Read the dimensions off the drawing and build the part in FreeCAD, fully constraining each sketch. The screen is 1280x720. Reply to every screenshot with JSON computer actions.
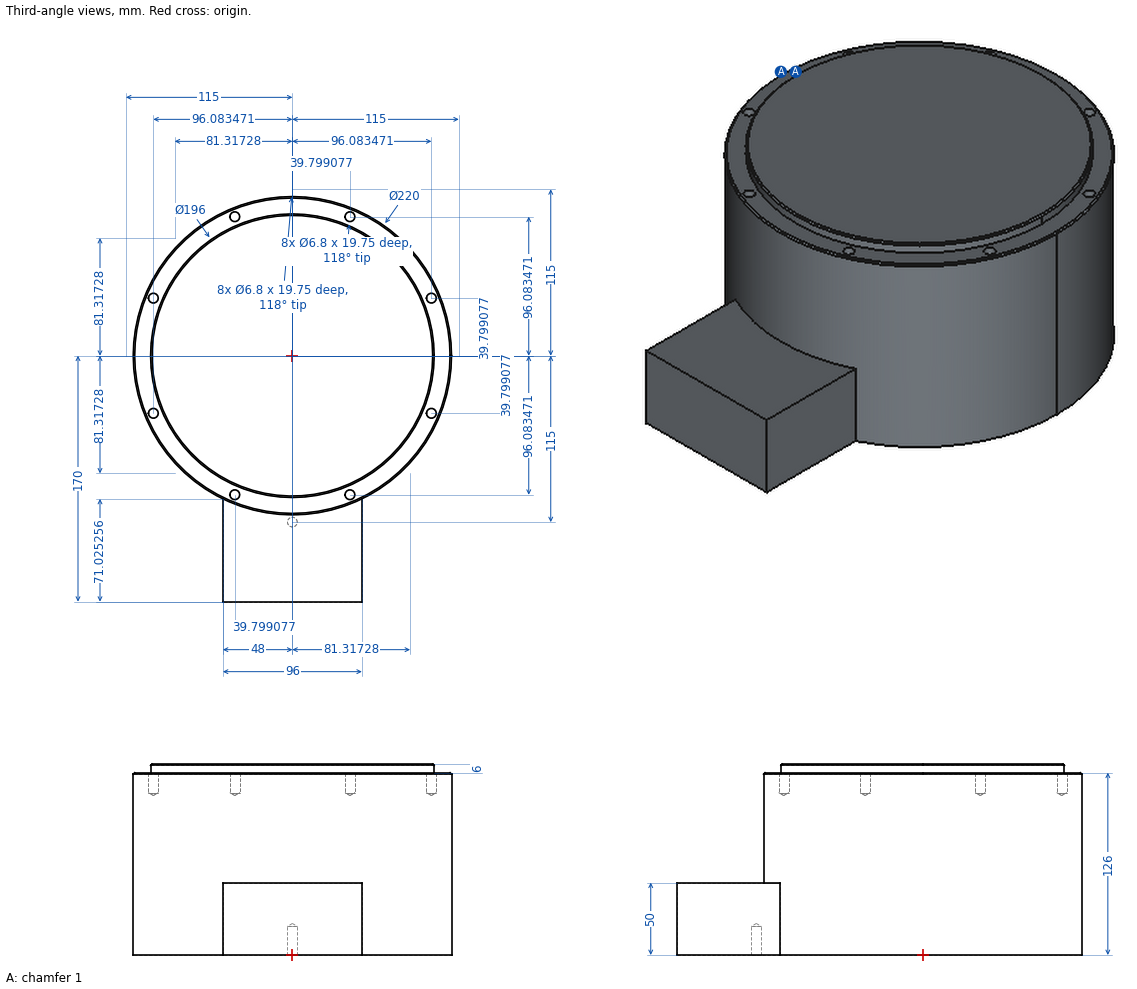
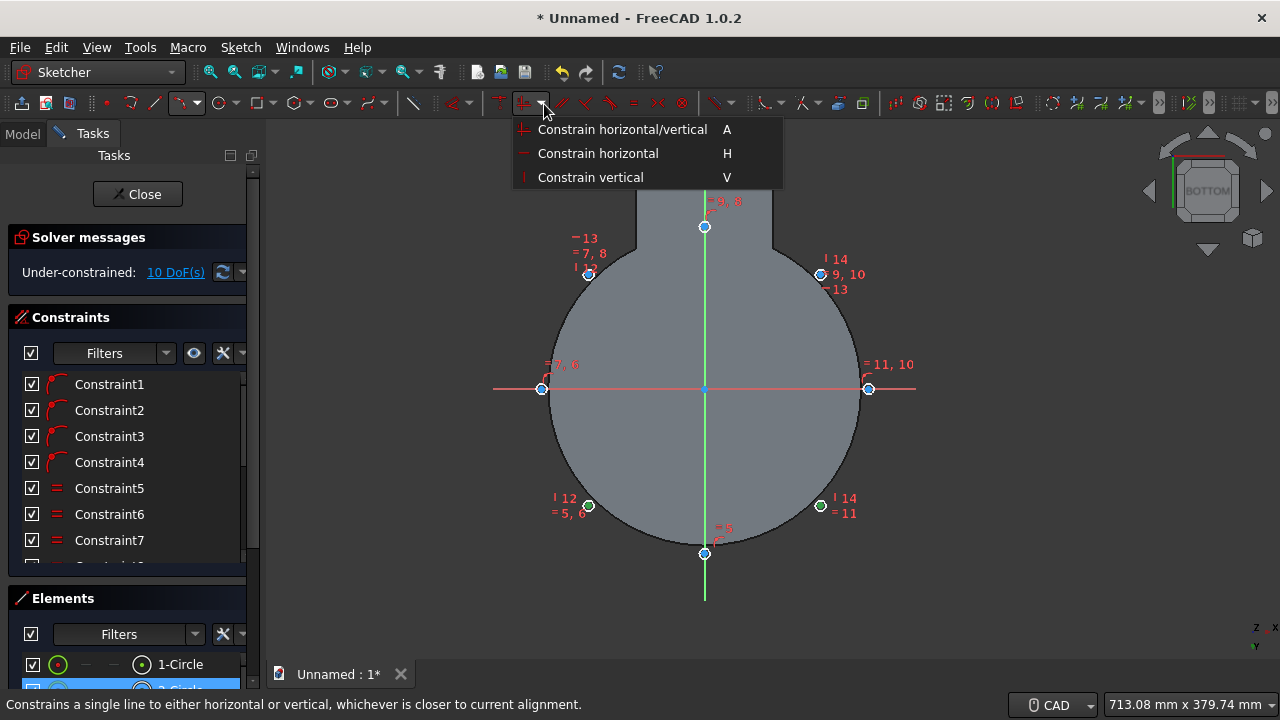
{"action": "left_click", "coordinate": [648, 153]}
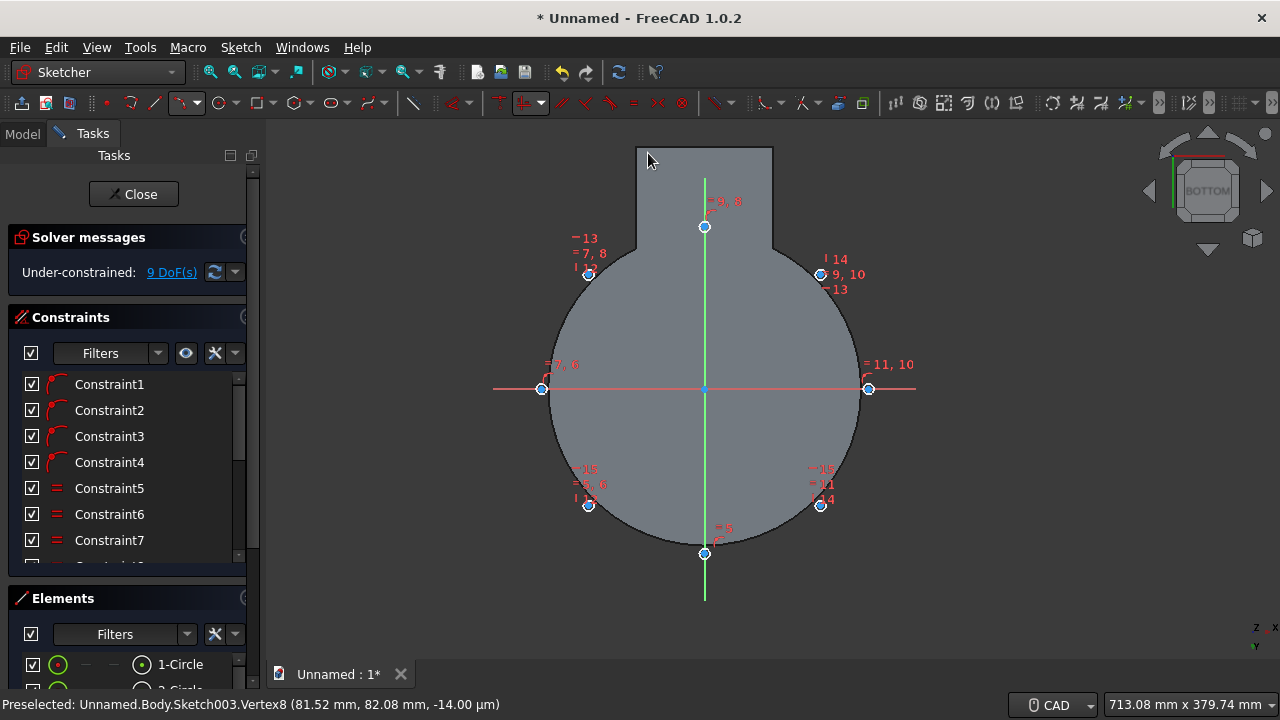
{"action": "left_click", "coordinate": [452, 104]}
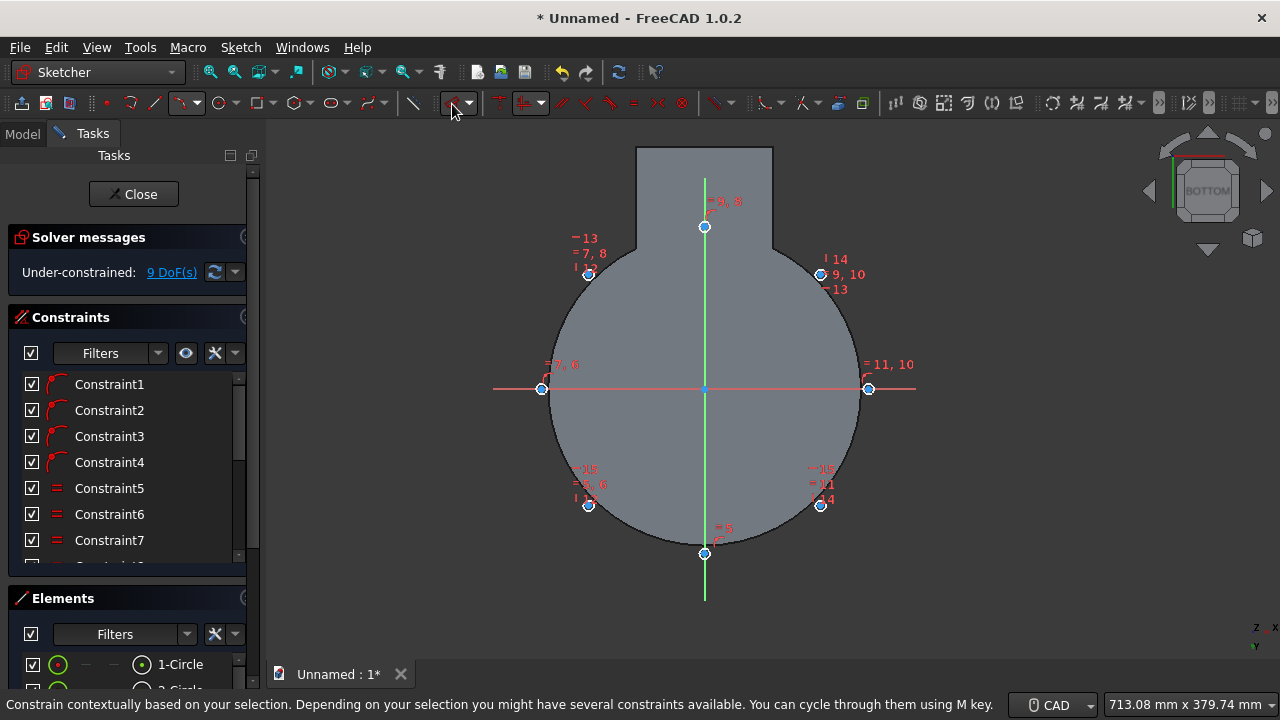
{"action": "scroll", "coordinate": [705, 549], "scroll_direction": "up", "scroll_amount": 8}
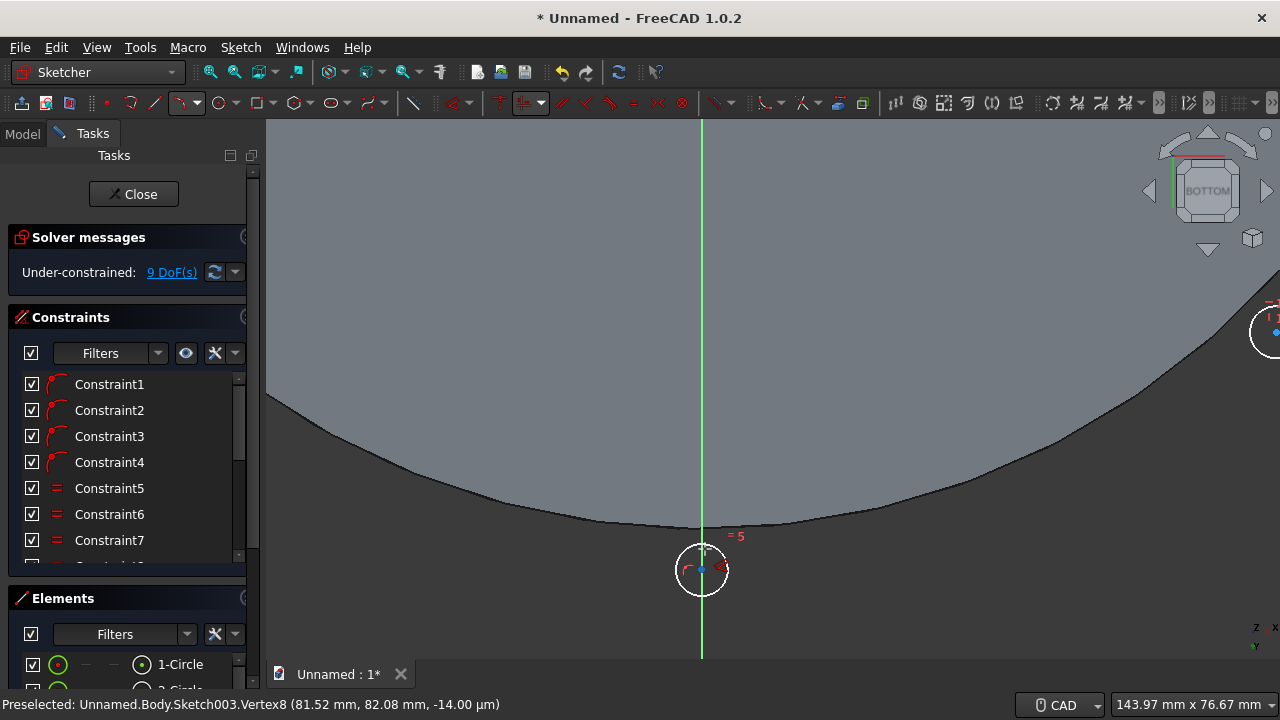
{"action": "left_click", "coordinate": [703, 544]}
{"action": "left_click", "coordinate": [732, 520]}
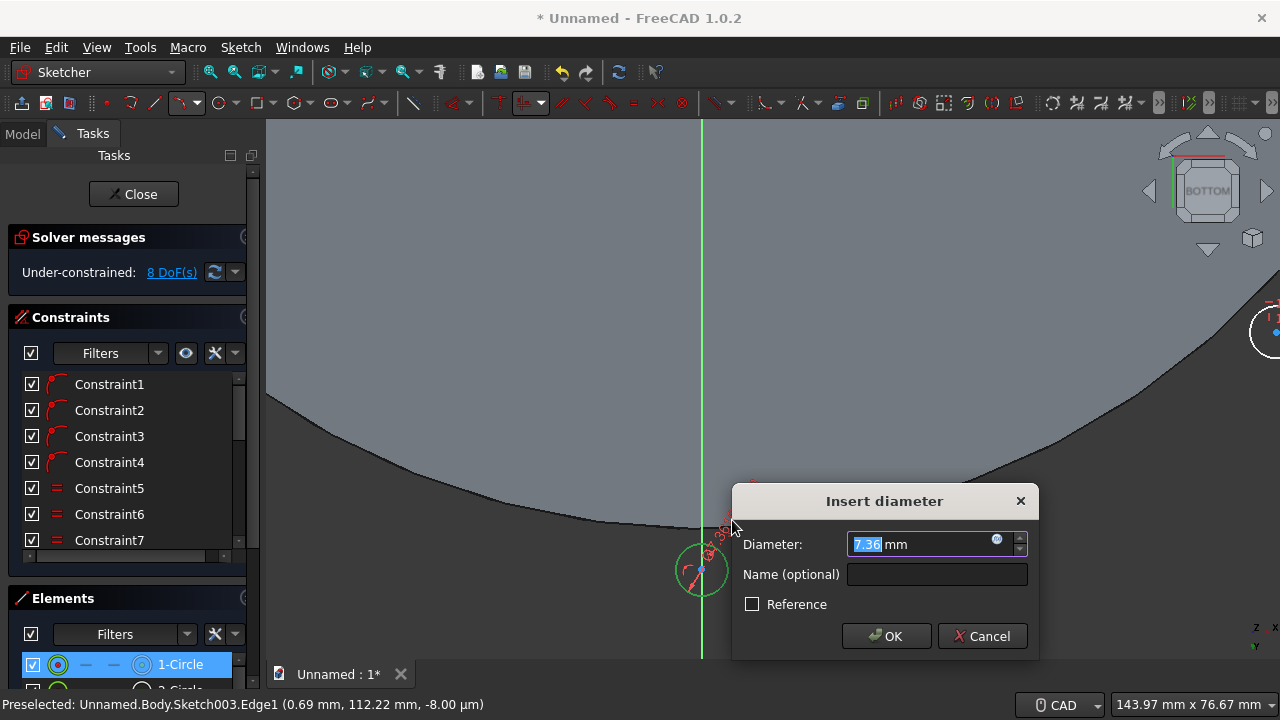
{"action": "type", "text": "6.8"}
{"action": "key", "text": "Return"}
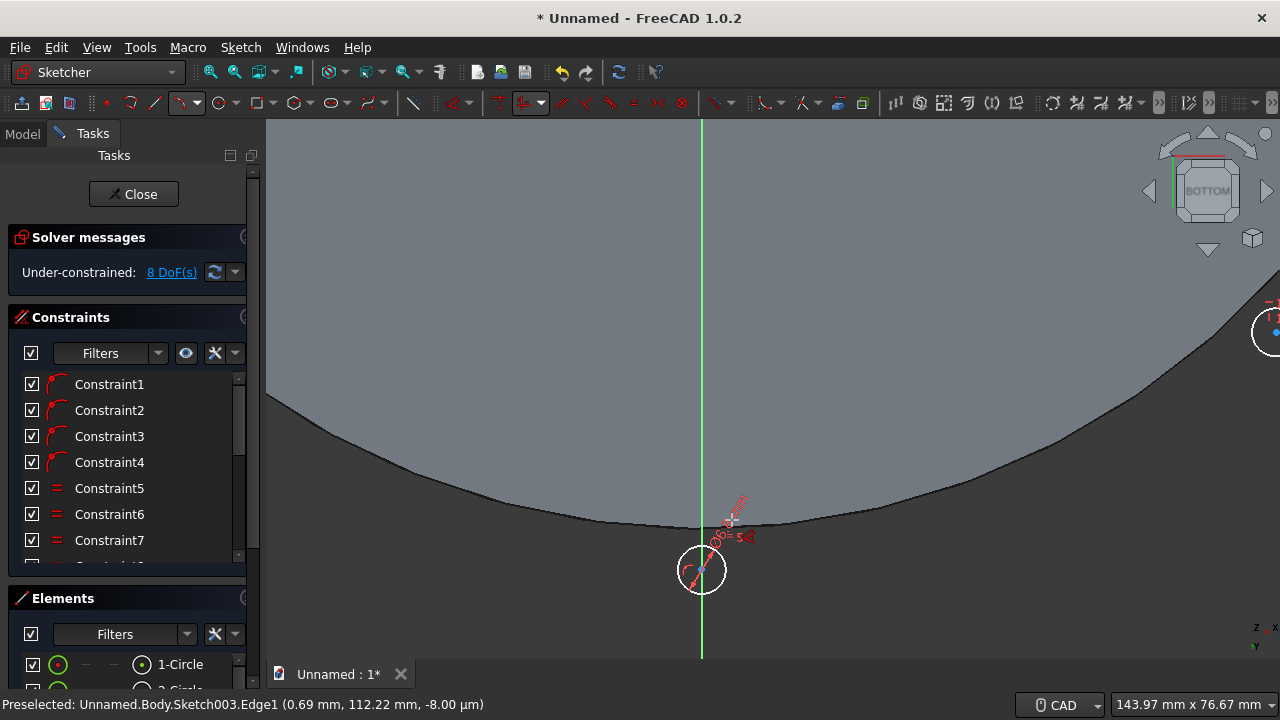
{"action": "scroll", "coordinate": [705, 550], "scroll_direction": "down", "scroll_amount": 8}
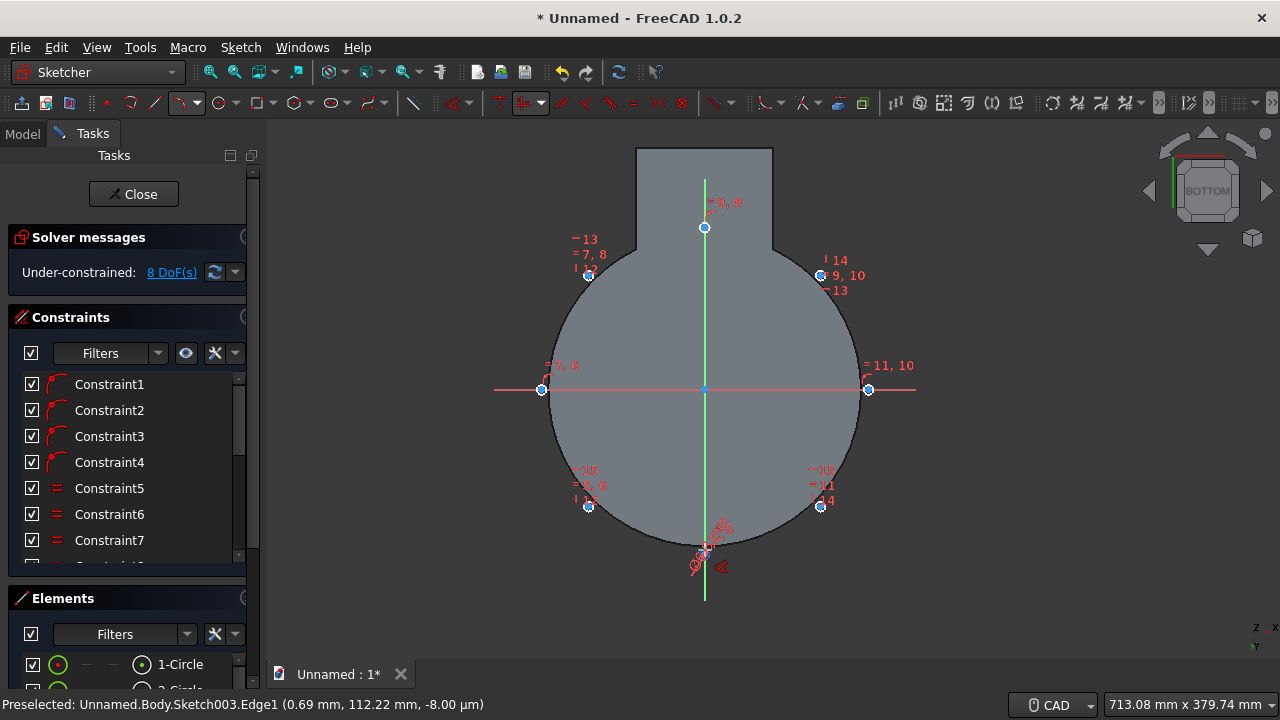
{"action": "left_click", "coordinate": [705, 555]}
{"action": "left_click", "coordinate": [739, 472]}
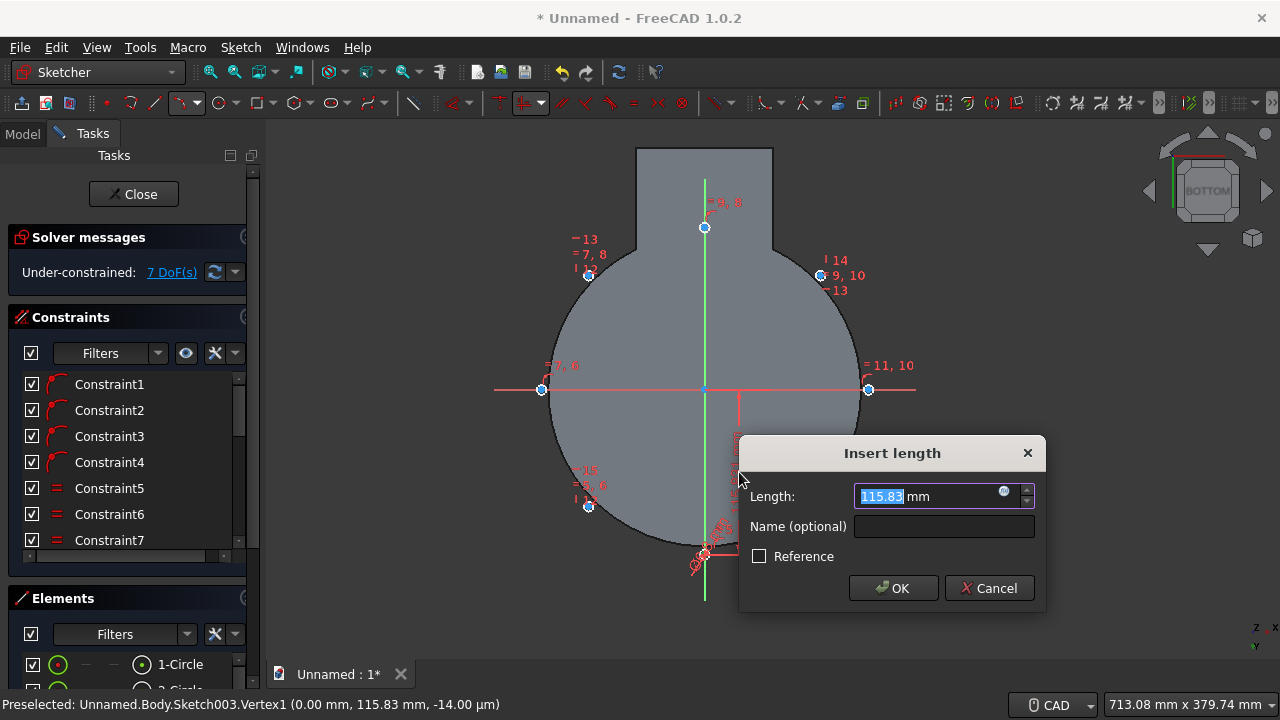
{"action": "type", "text": "115"}
{"action": "key", "text": "Return"}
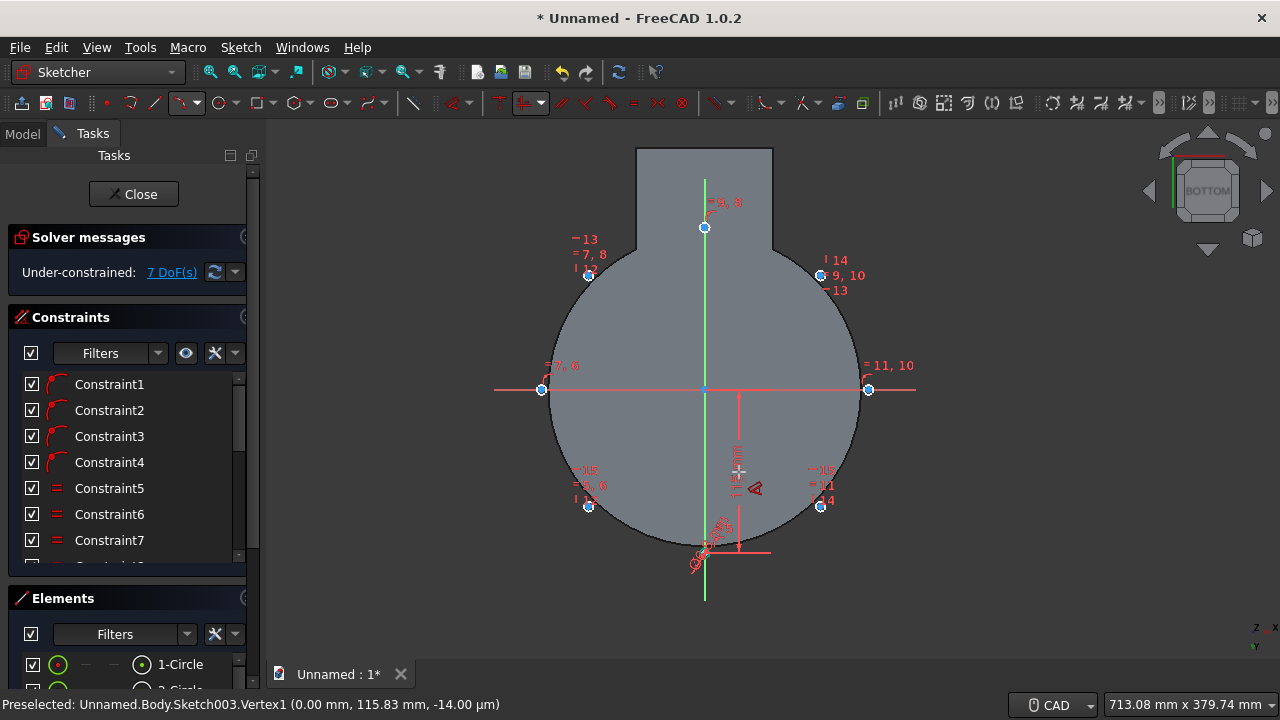
{"action": "left_click", "coordinate": [542, 390]}
{"action": "left_click", "coordinate": [623, 424]}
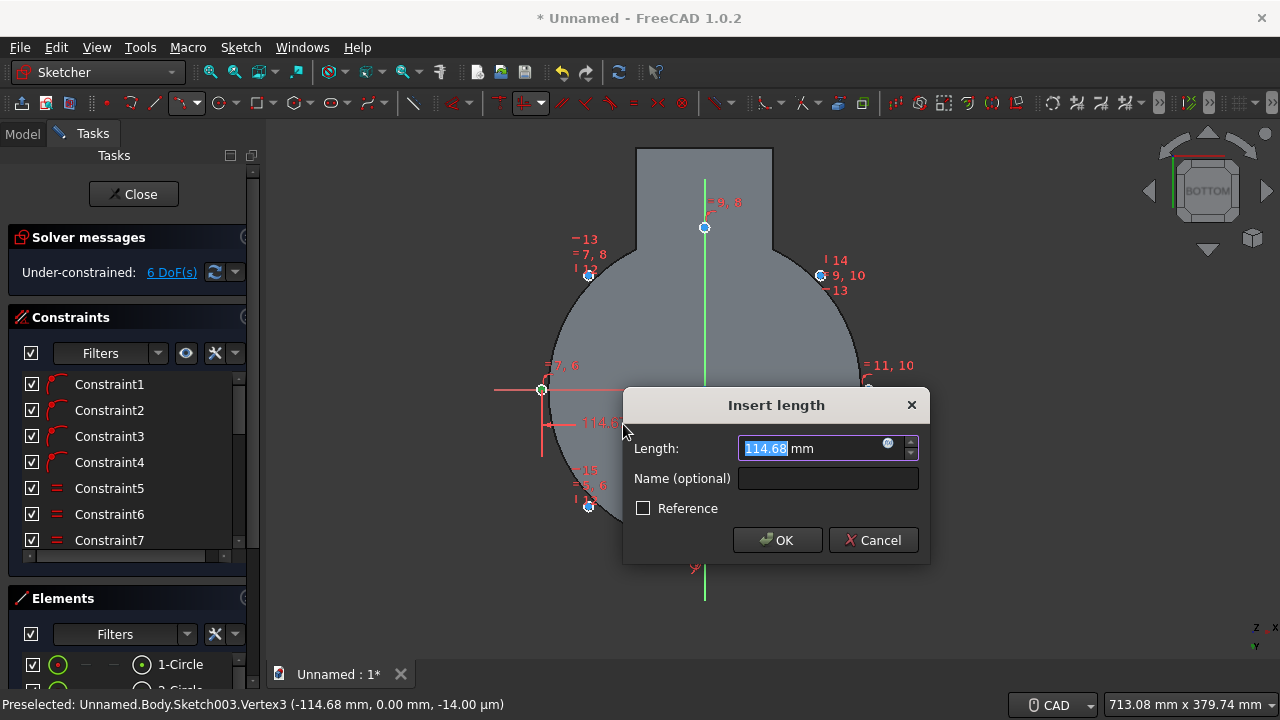
{"action": "type", "text": "115"}
{"action": "key", "text": "Return"}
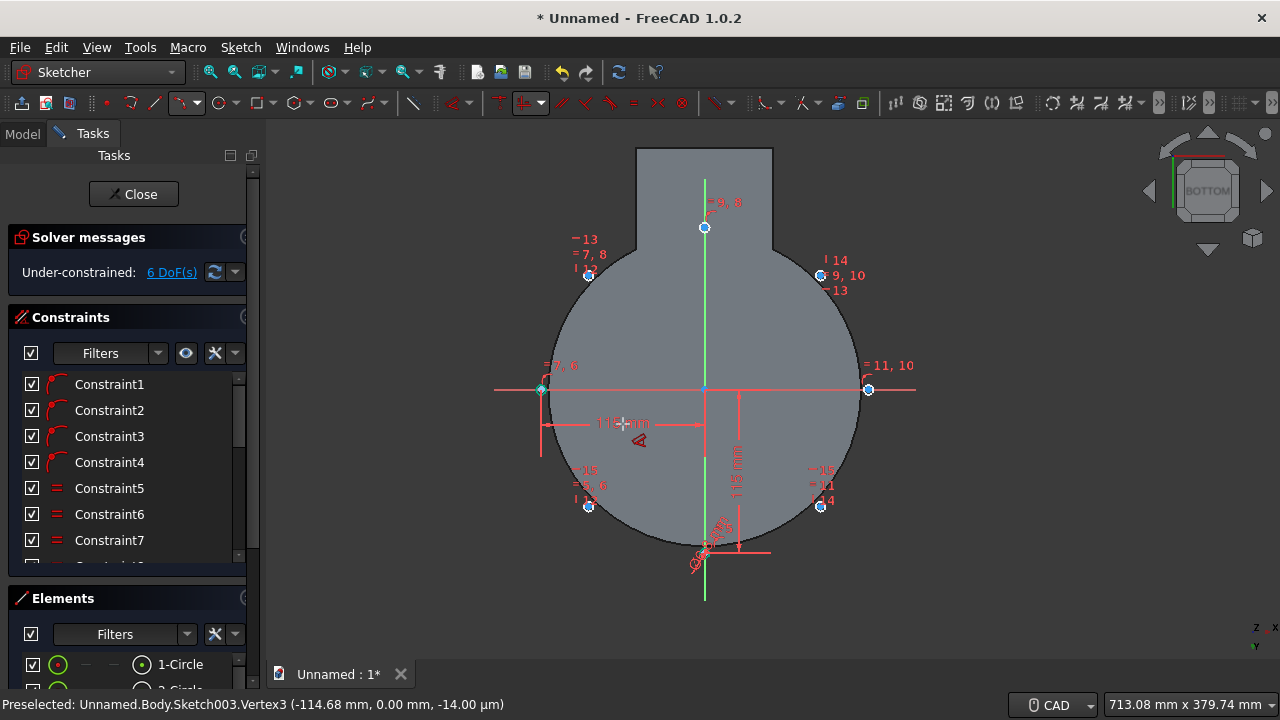
{"action": "left_click", "coordinate": [705, 228]}
{"action": "left_click", "coordinate": [739, 309]}